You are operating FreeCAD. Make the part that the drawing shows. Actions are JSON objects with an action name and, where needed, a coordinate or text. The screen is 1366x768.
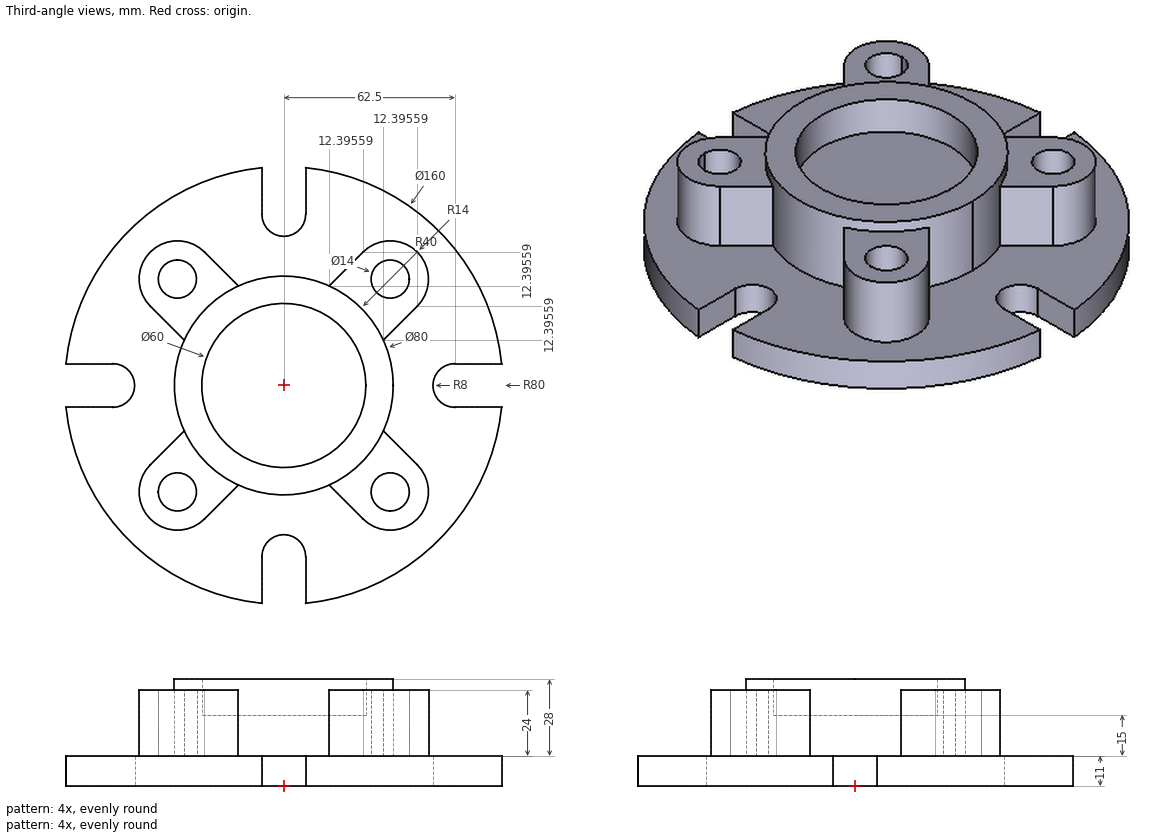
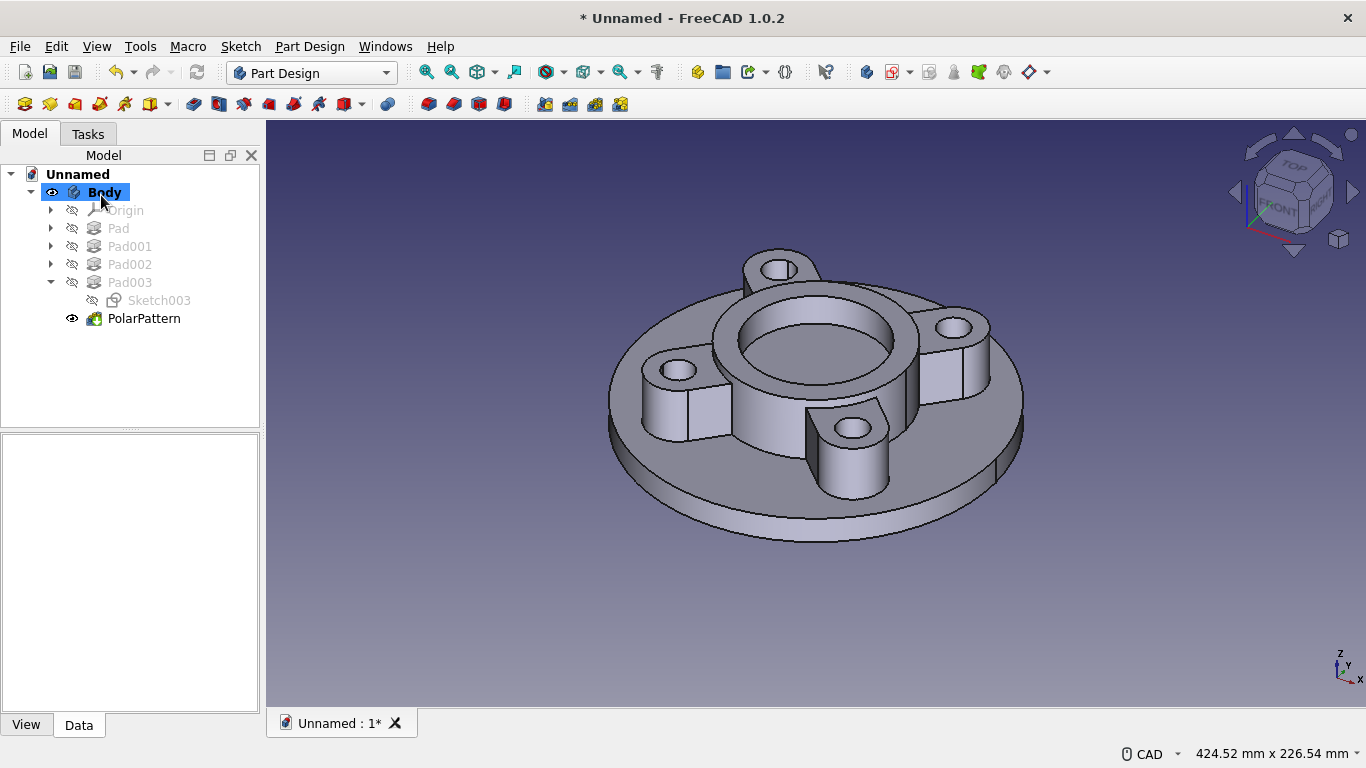
{"action": "left_click", "coordinate": [51, 210]}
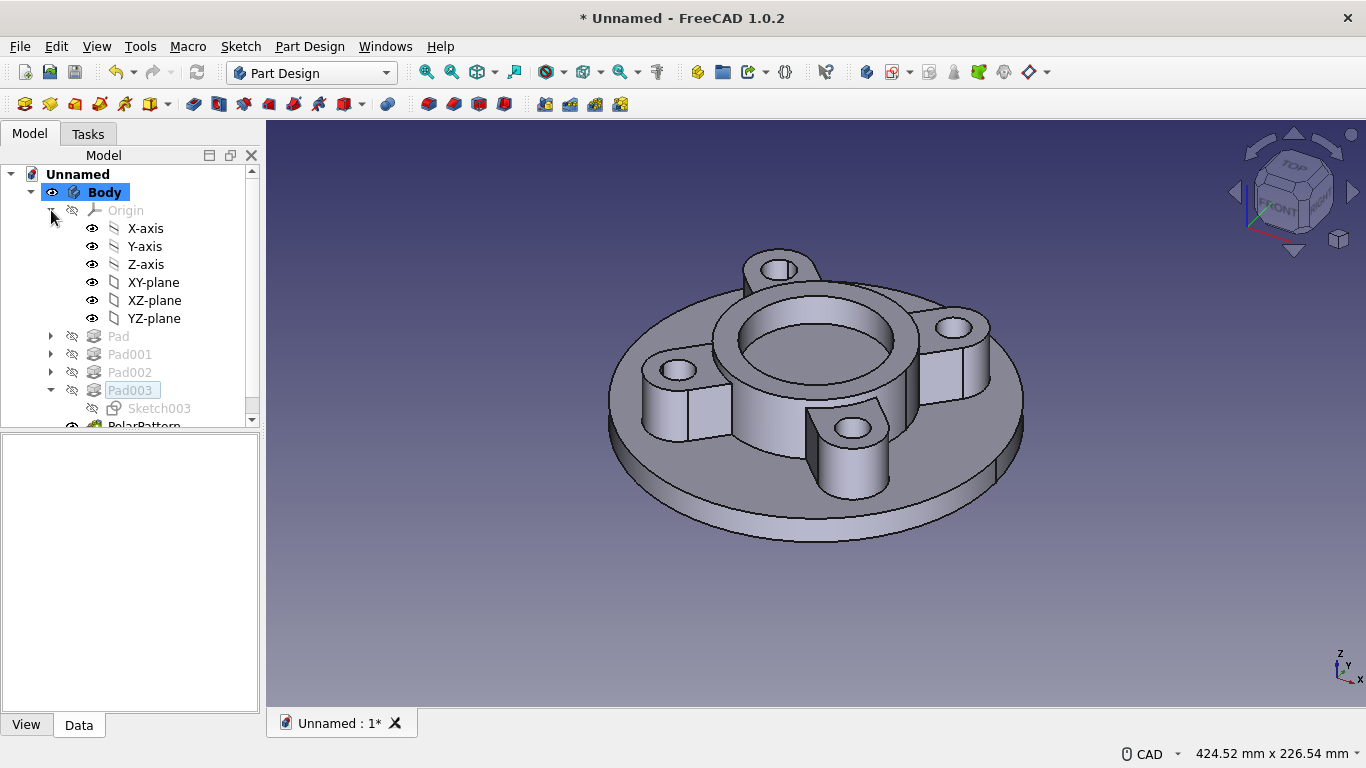
{"action": "left_click", "coordinate": [137, 282]}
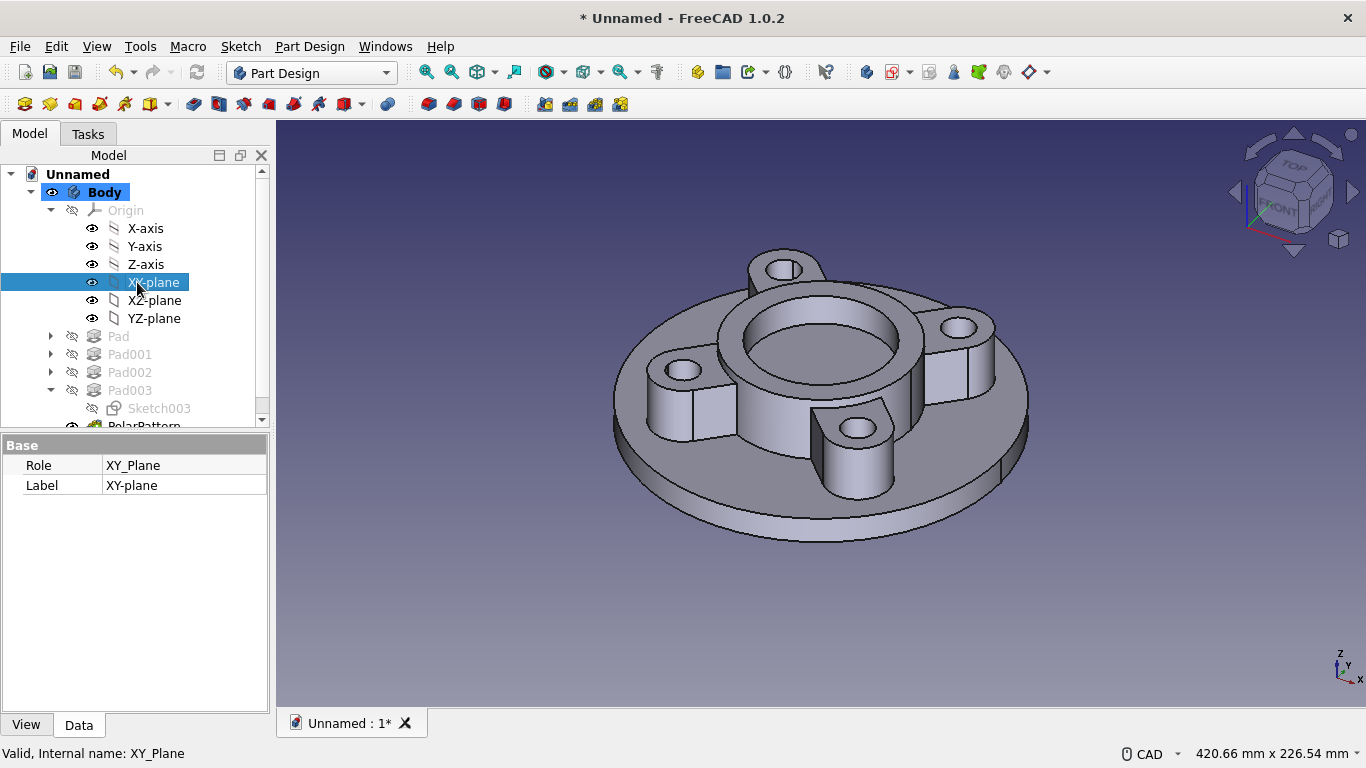
{"action": "left_click", "coordinate": [1028, 72]}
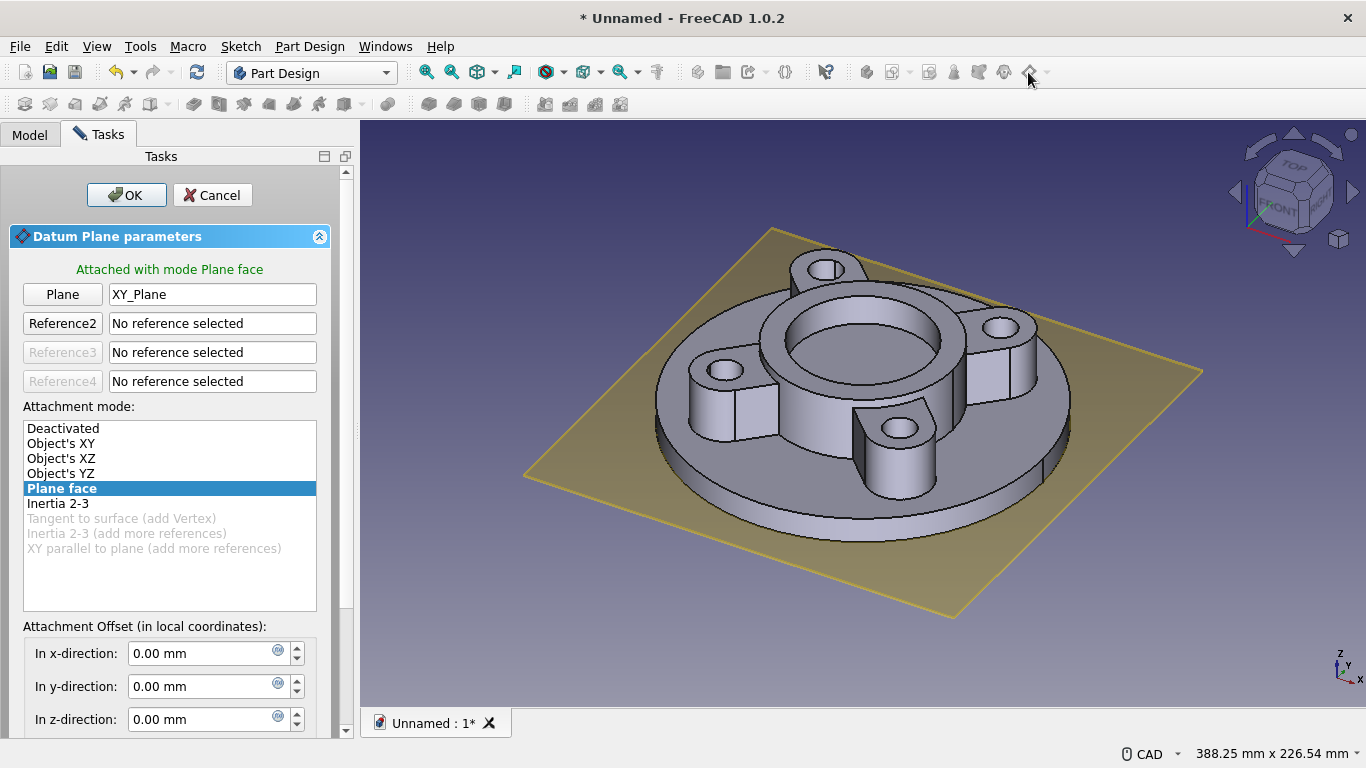
{"action": "triple_click", "coordinate": [210, 720]}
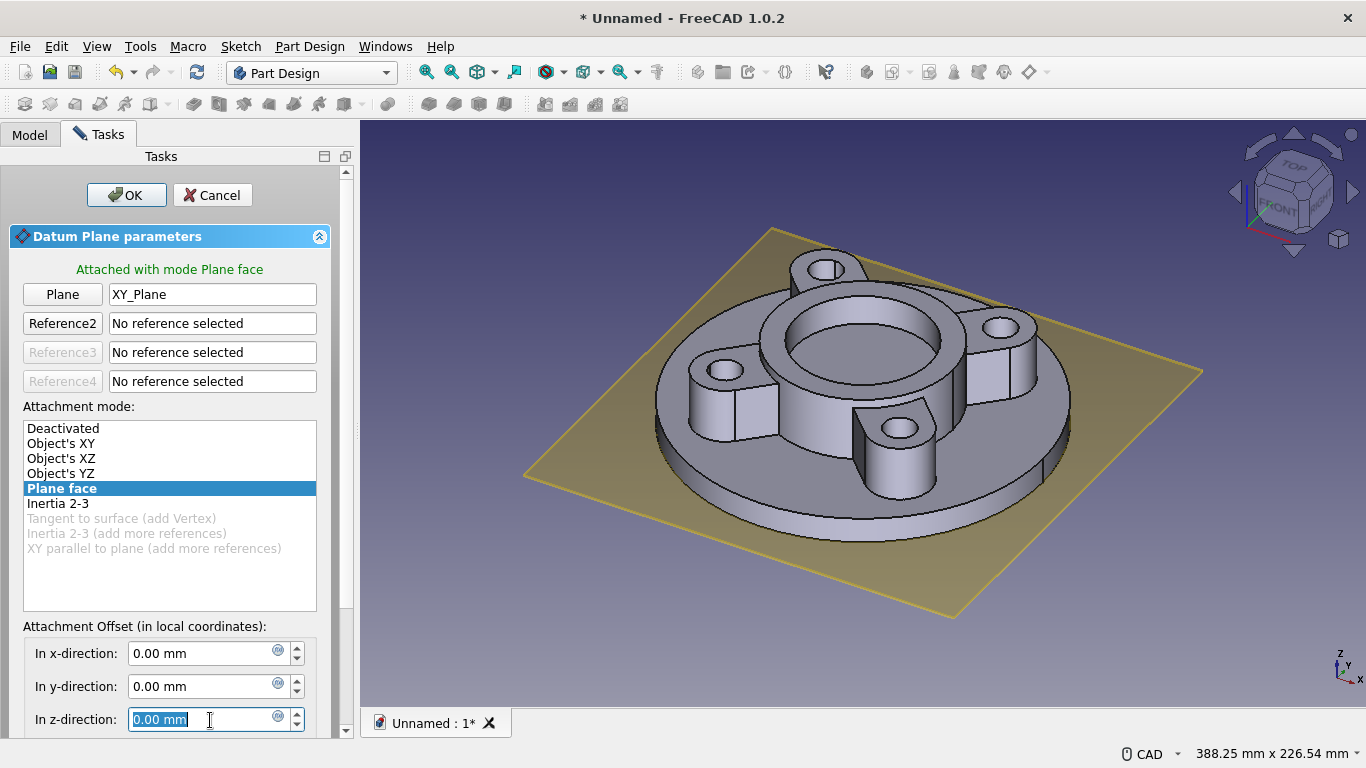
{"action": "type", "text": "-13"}
{"action": "key", "text": "Tab"}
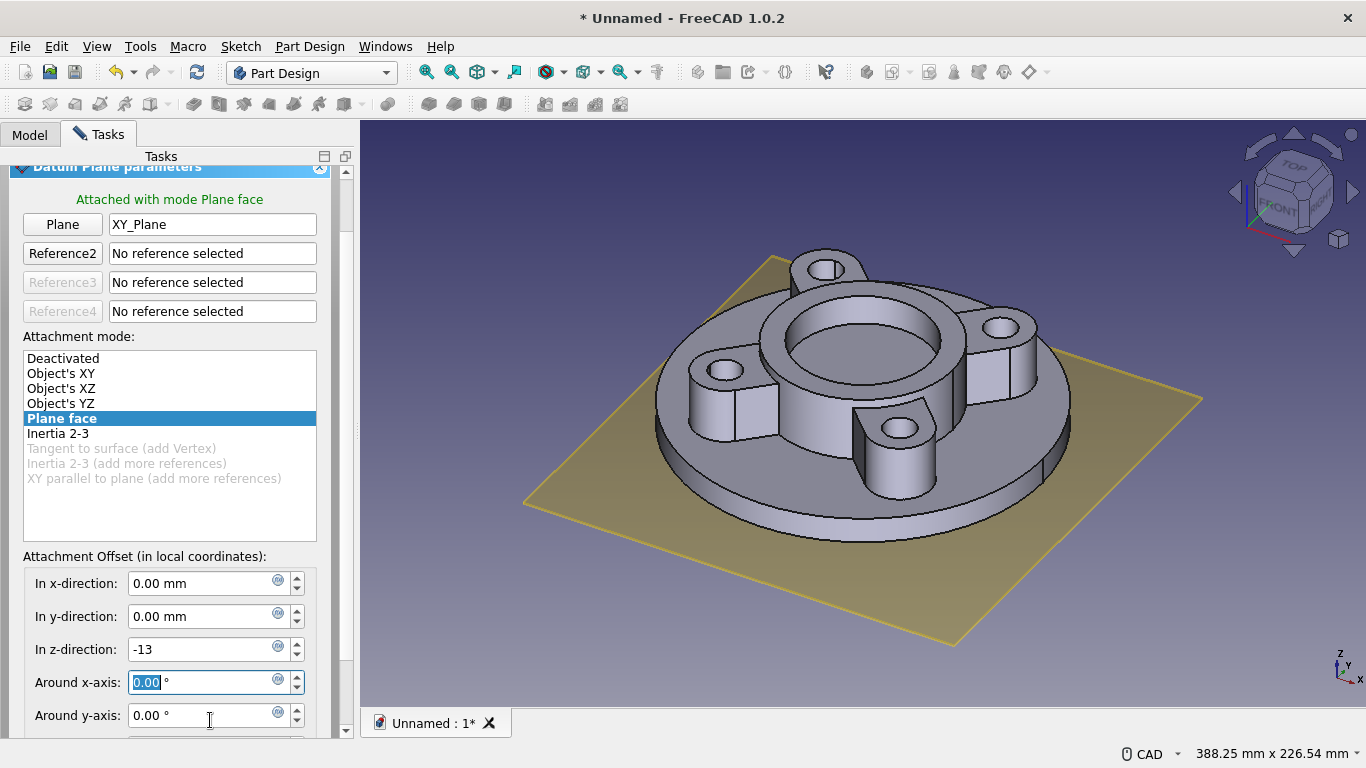
{"action": "scroll", "coordinate": [346, 452], "scroll_direction": "up", "scroll_amount": 2}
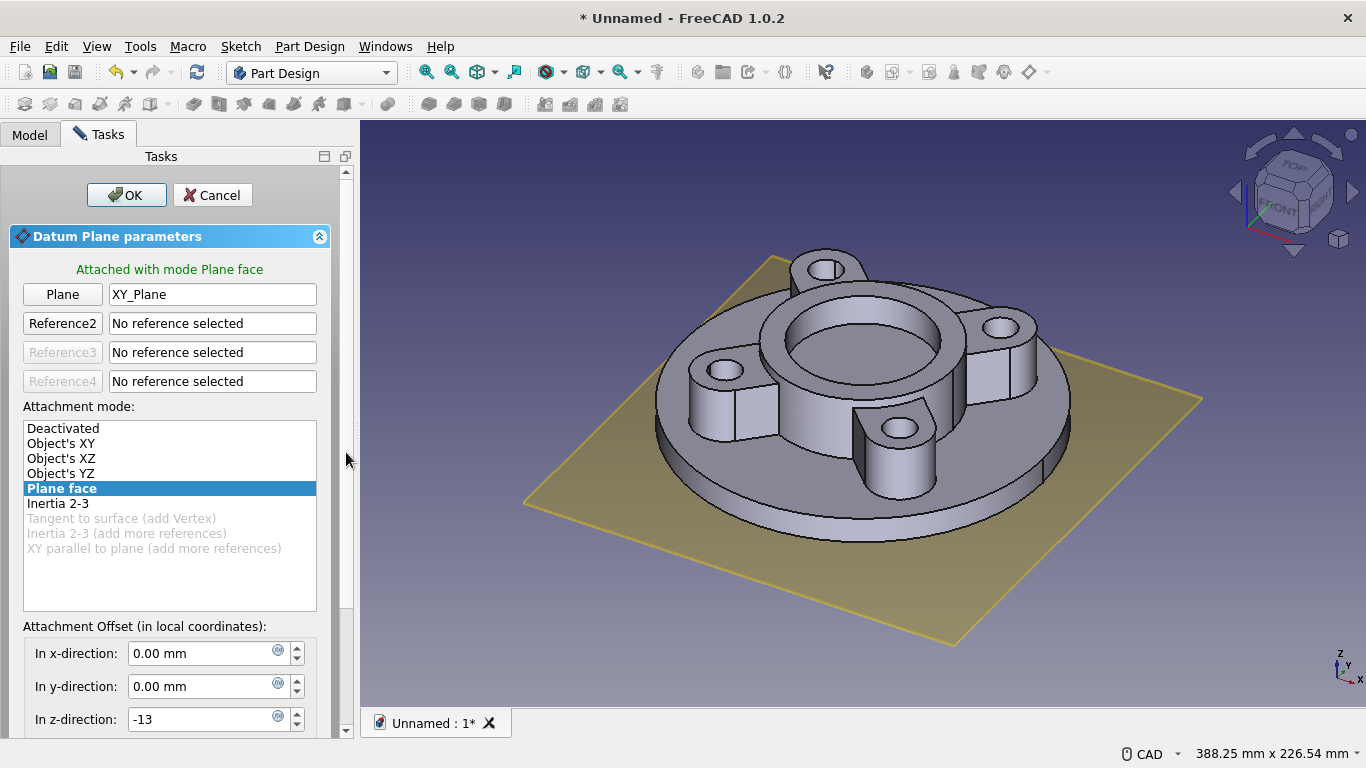
{"action": "left_click", "coordinate": [127, 195]}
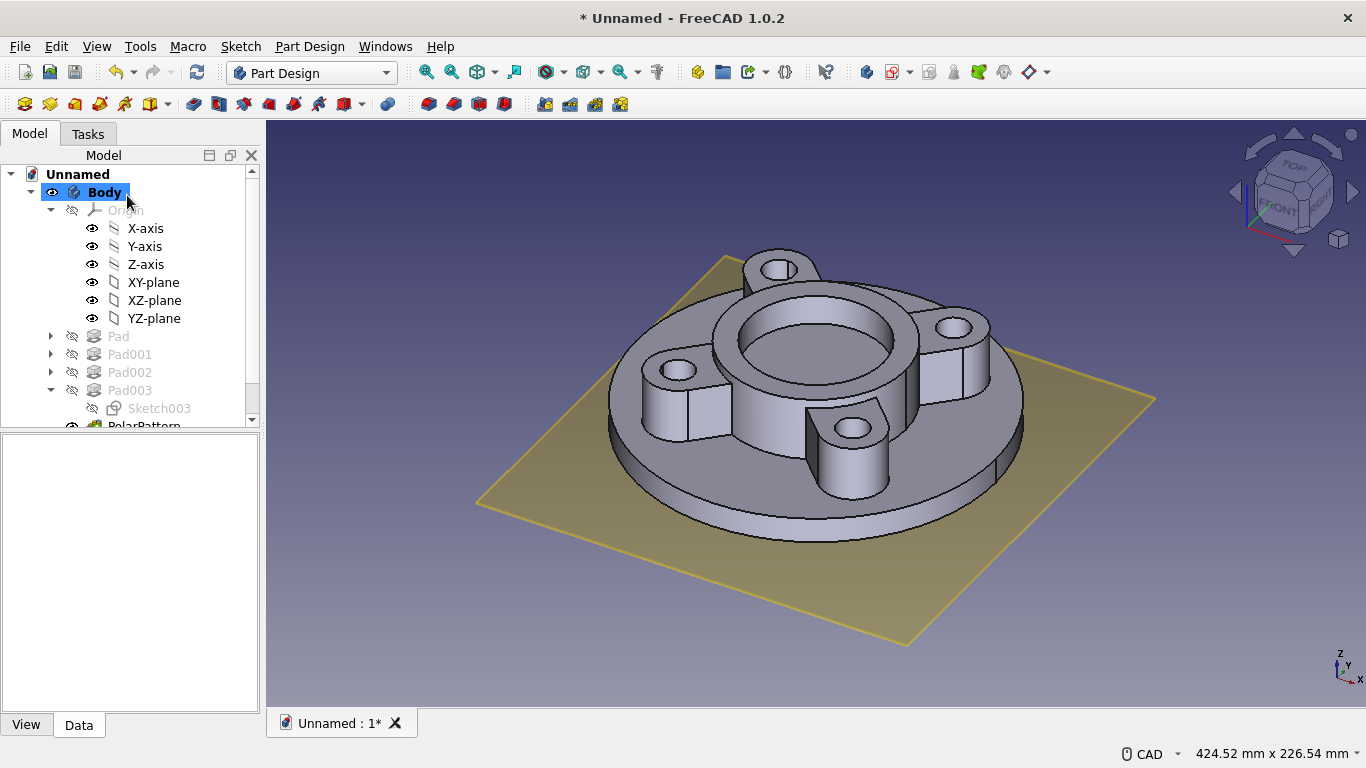
{"action": "scroll", "coordinate": [101, 296], "scroll_direction": "down", "scroll_amount": 3}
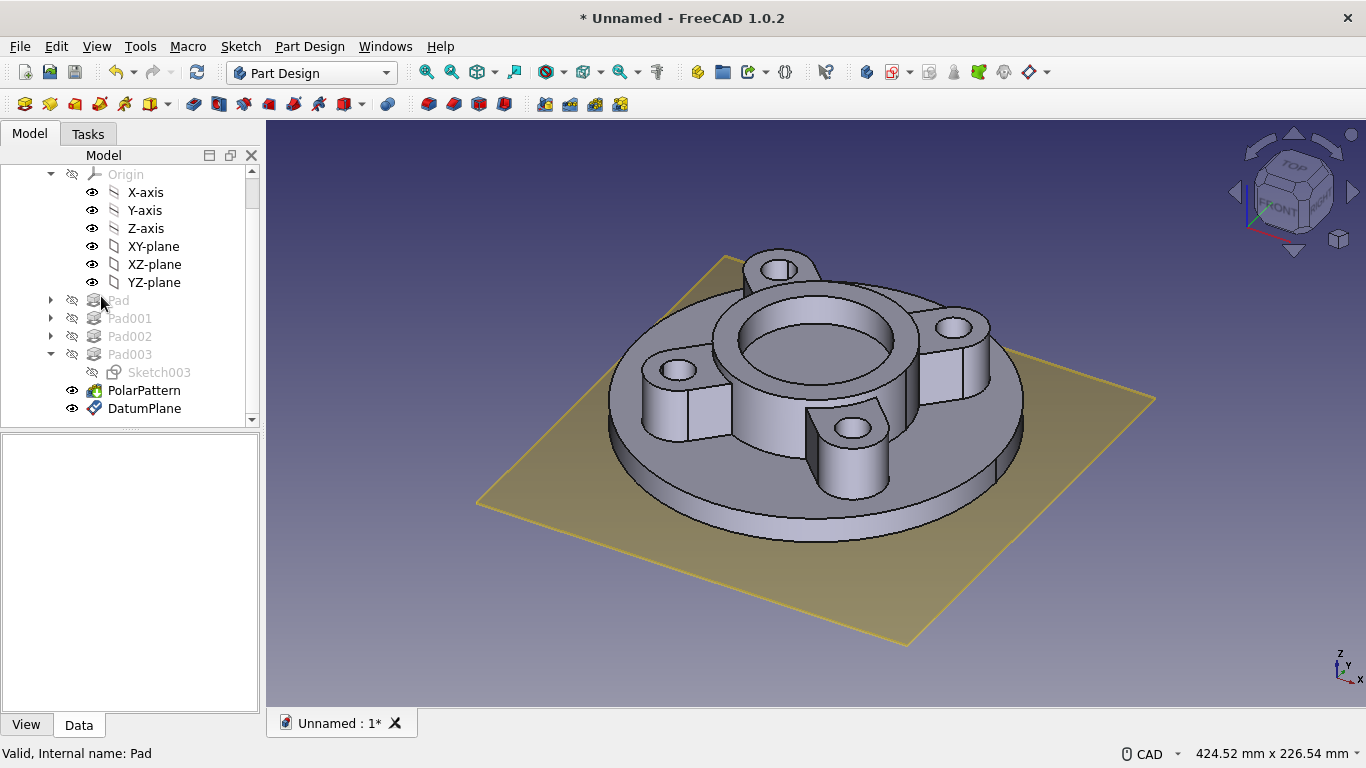
{"action": "left_click", "coordinate": [117, 408]}